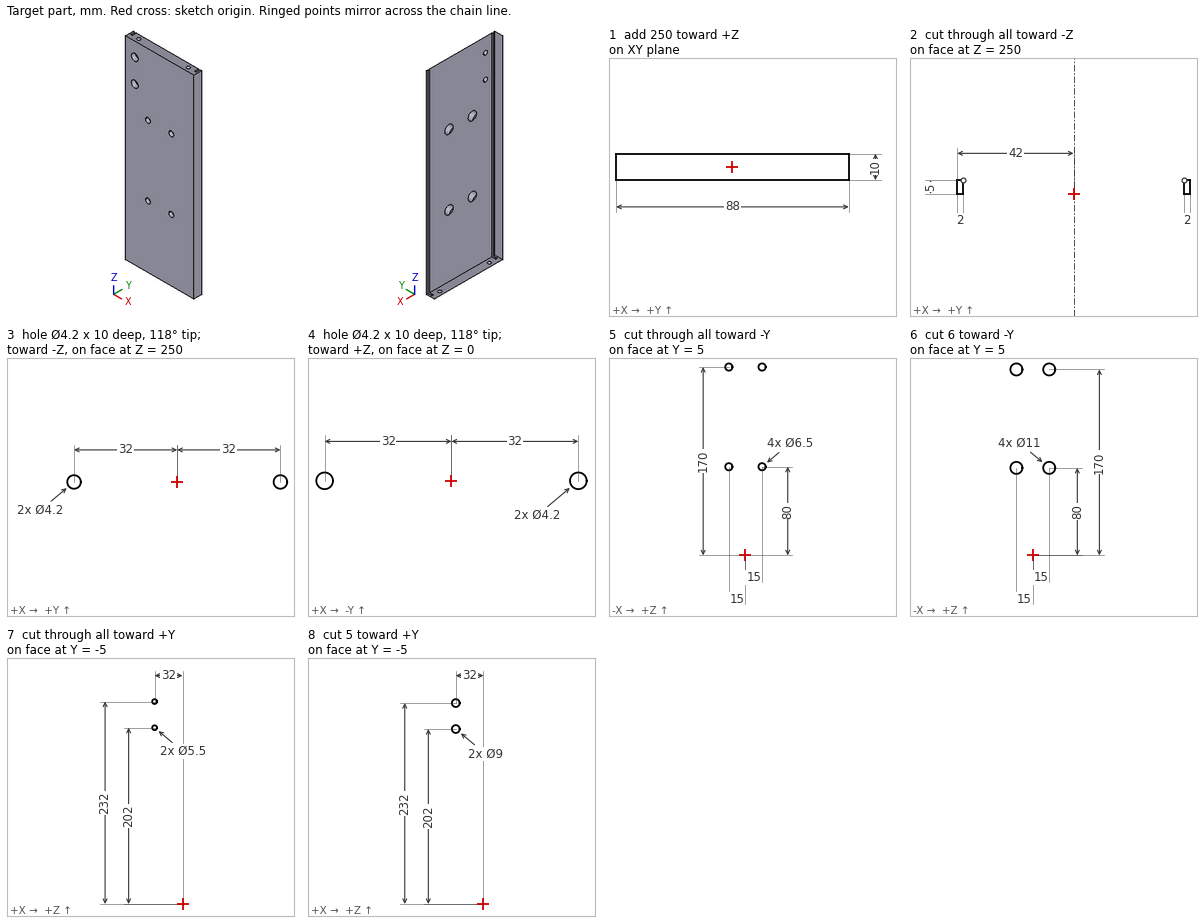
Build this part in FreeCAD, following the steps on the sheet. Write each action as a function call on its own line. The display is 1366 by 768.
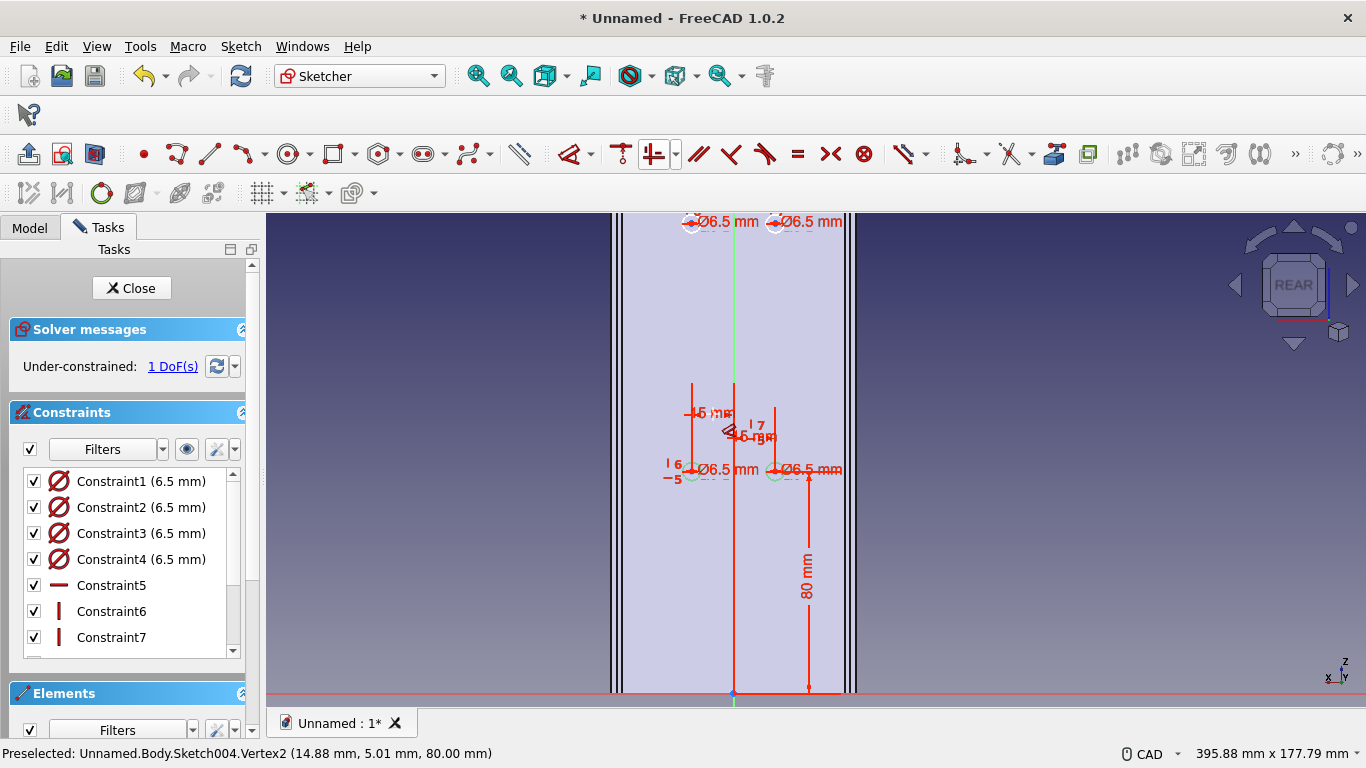
scroll(776, 474, down, 2)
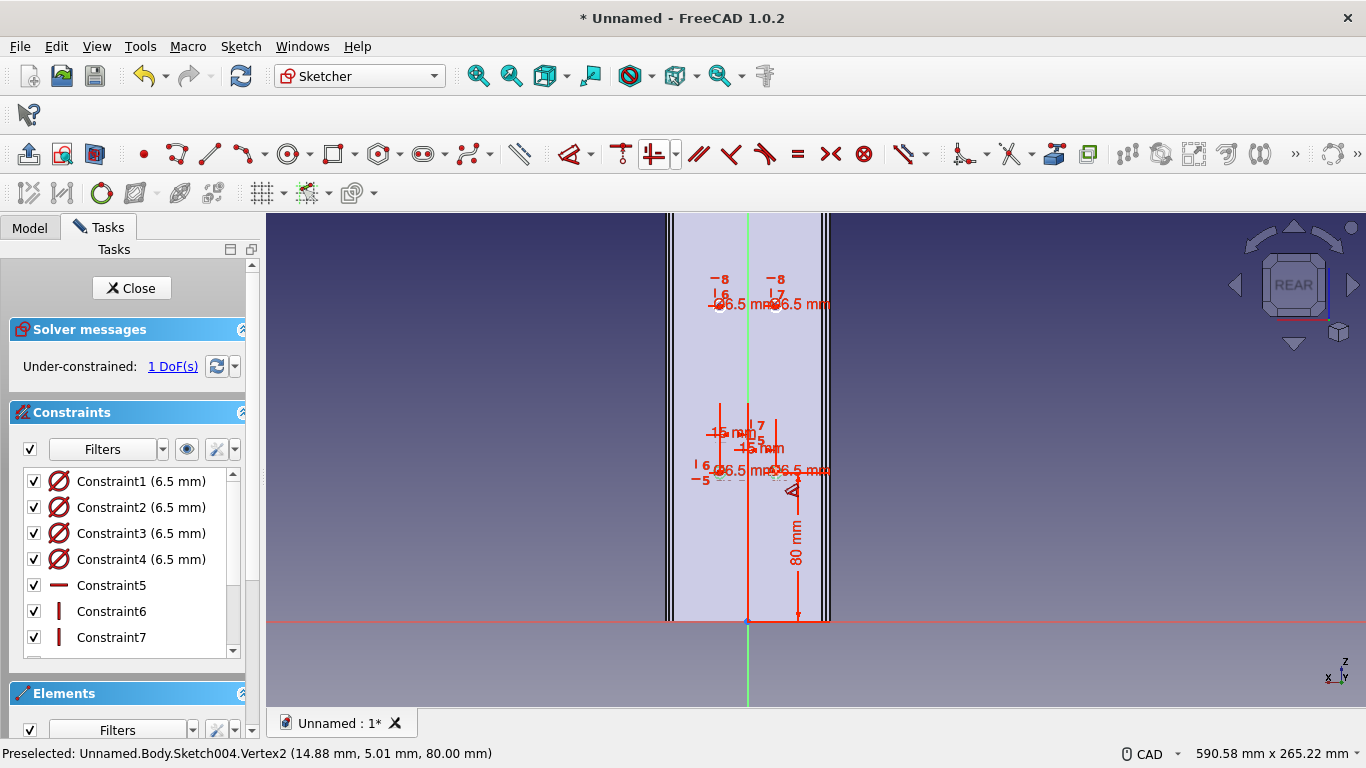
click(720, 306)
click(686, 464)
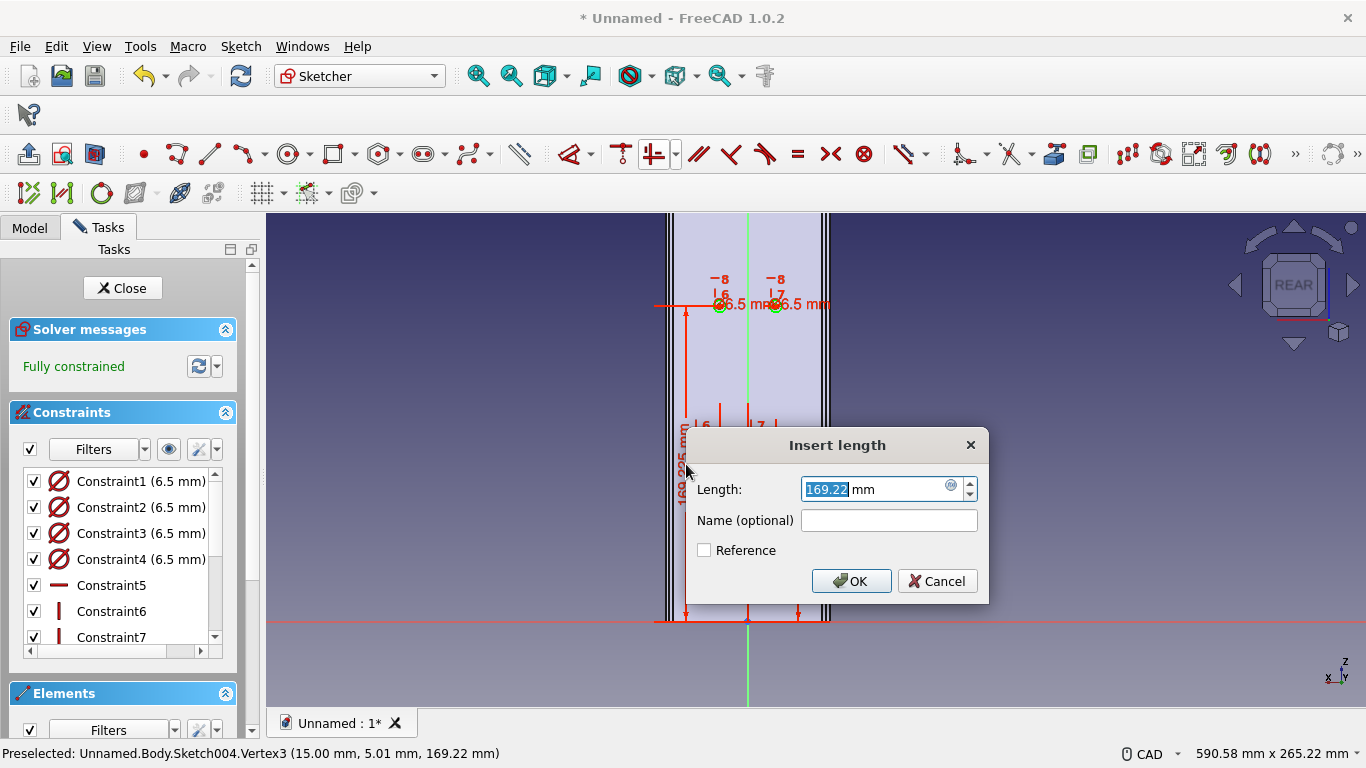
text(170)
key(Return)
key(Escape)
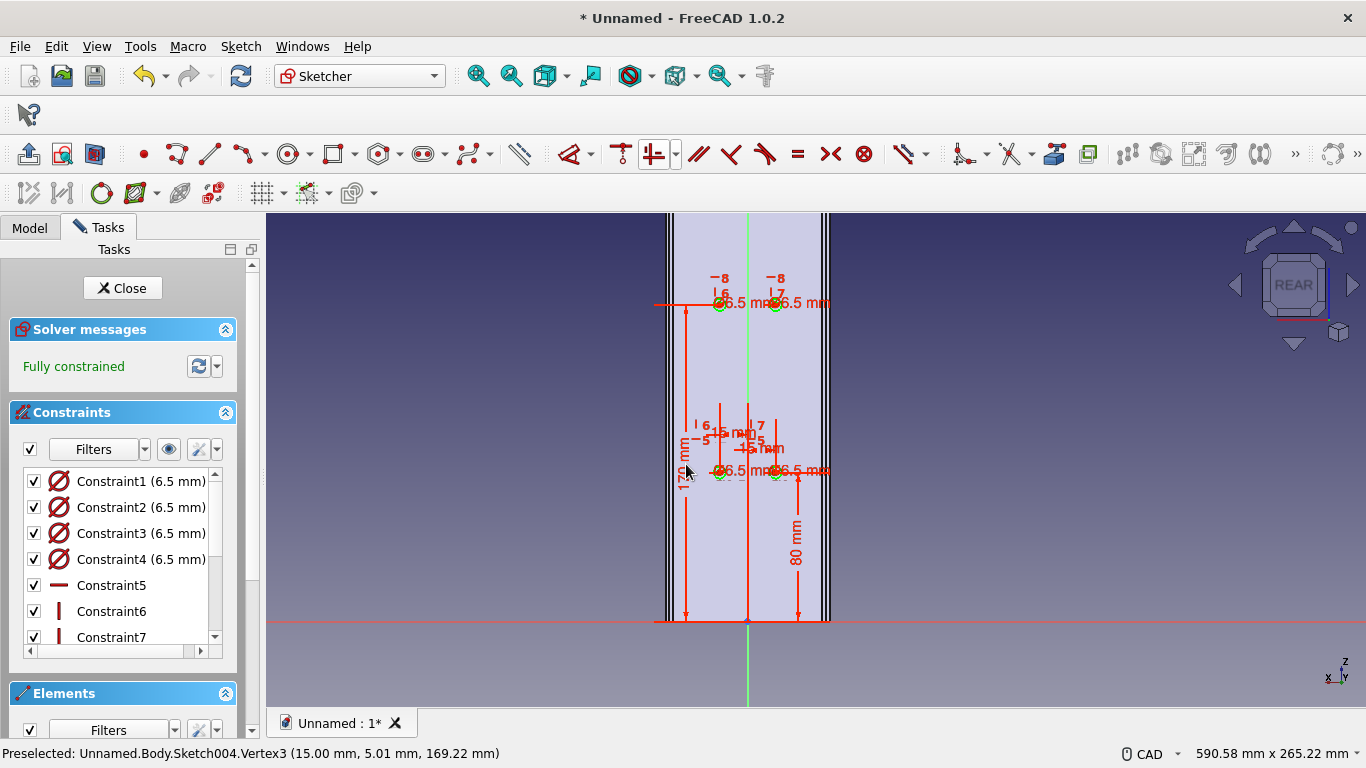
click(123, 288)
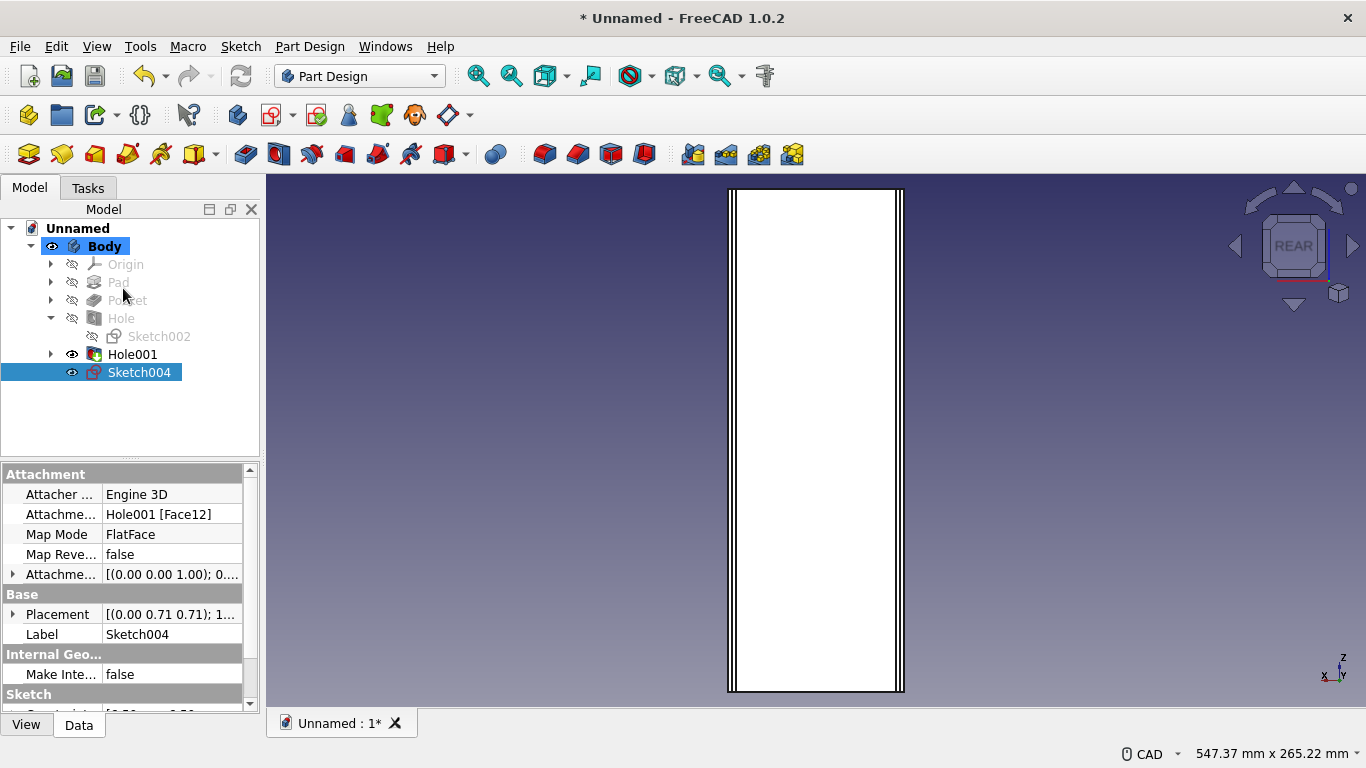
click(246, 154)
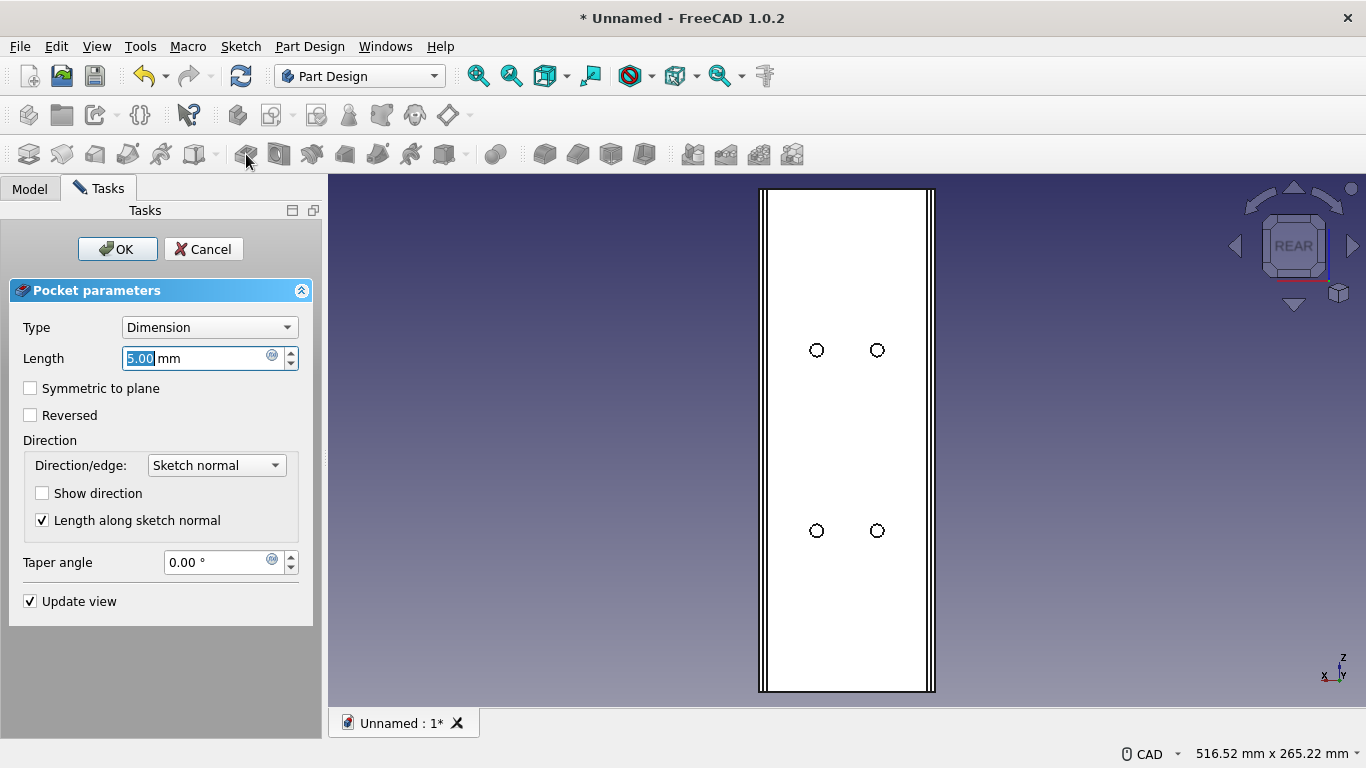
click(210, 328)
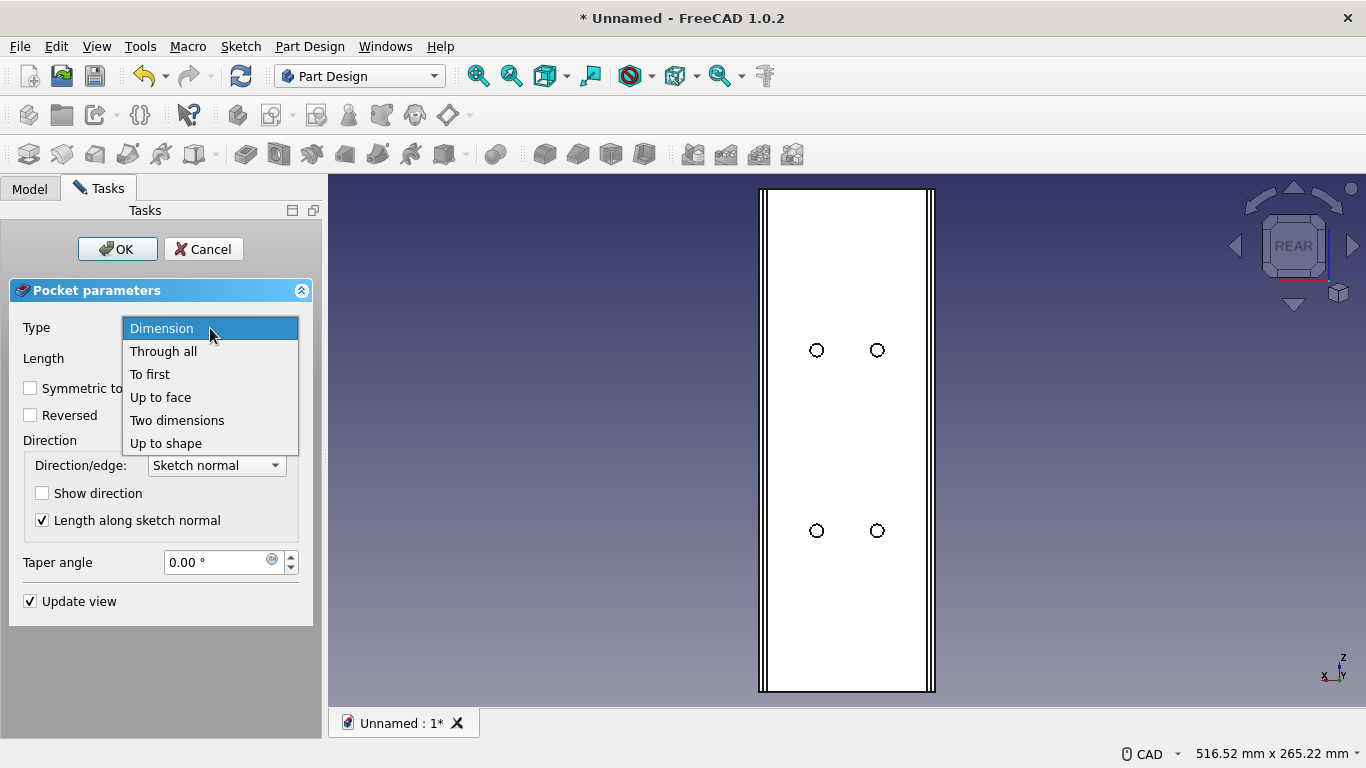
click(208, 352)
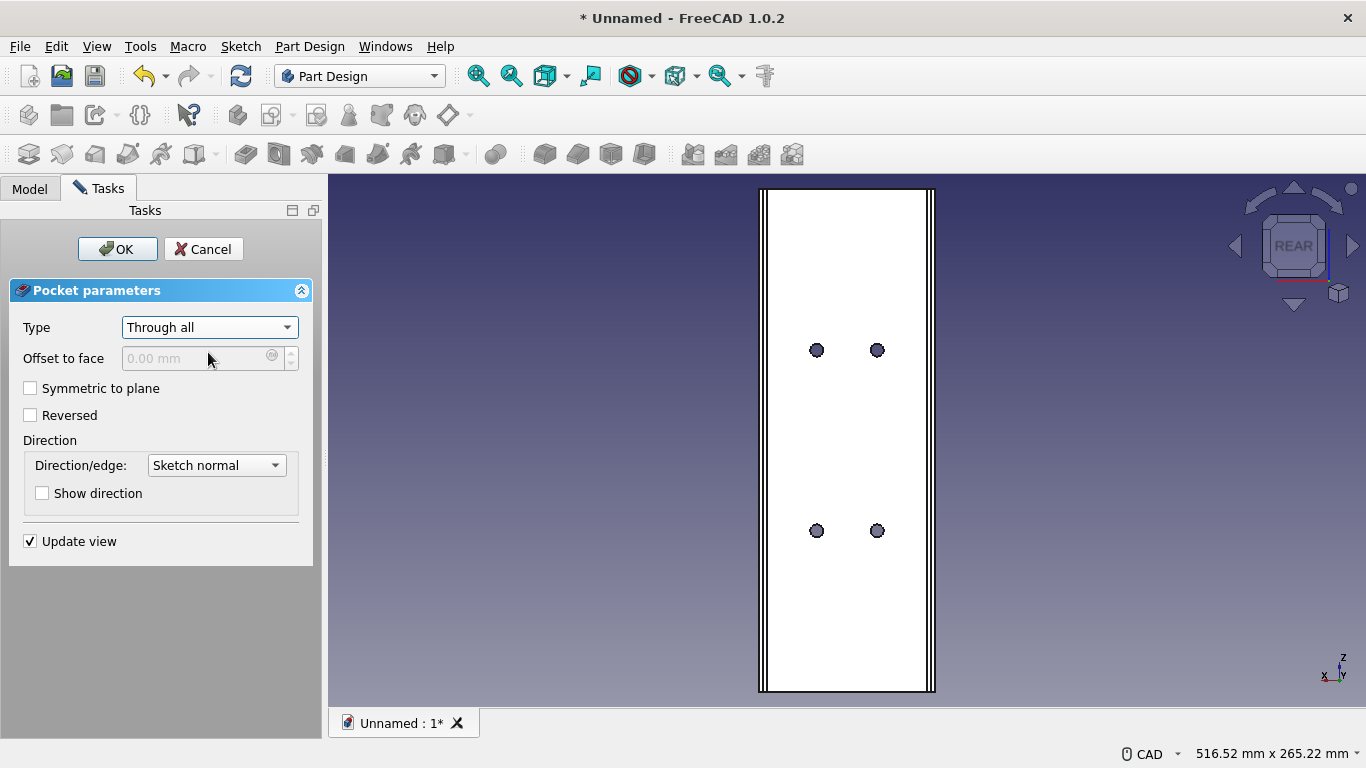
click(118, 249)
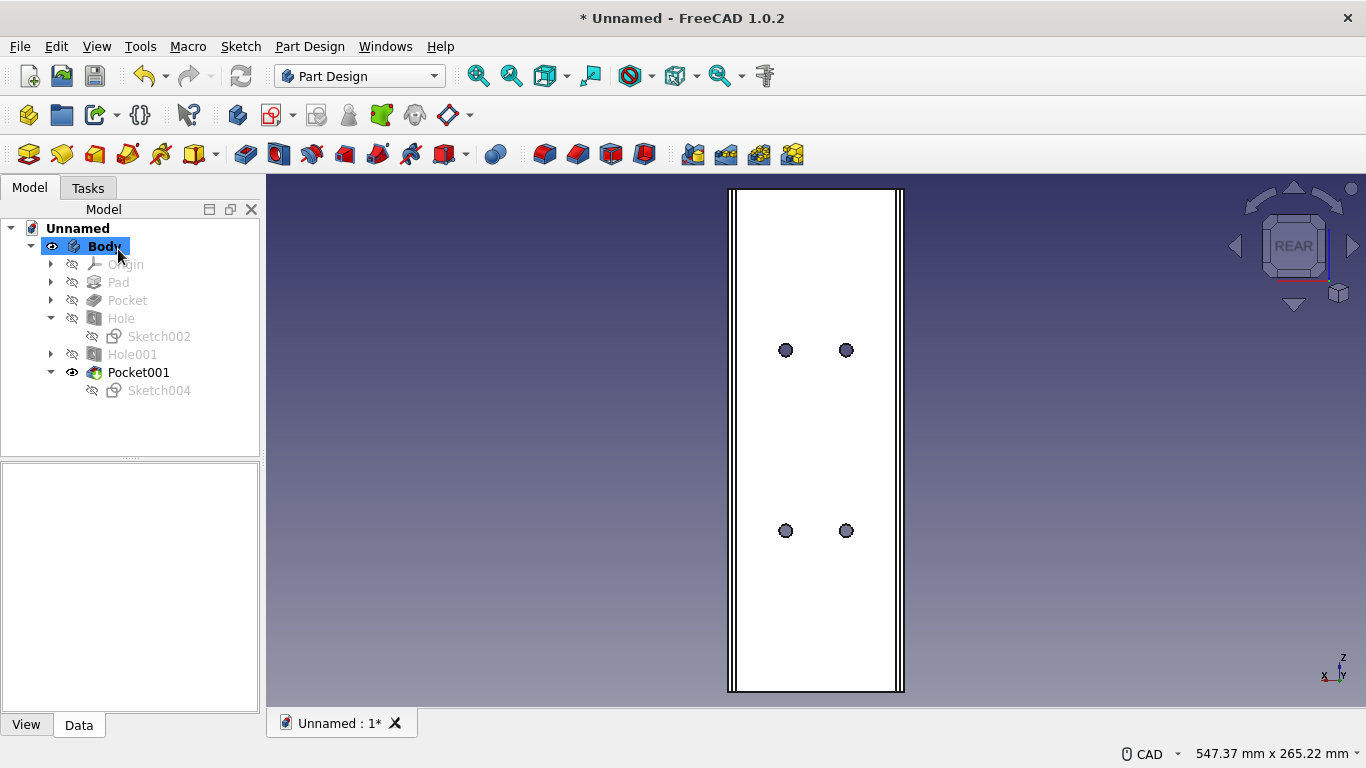
click(816, 439)